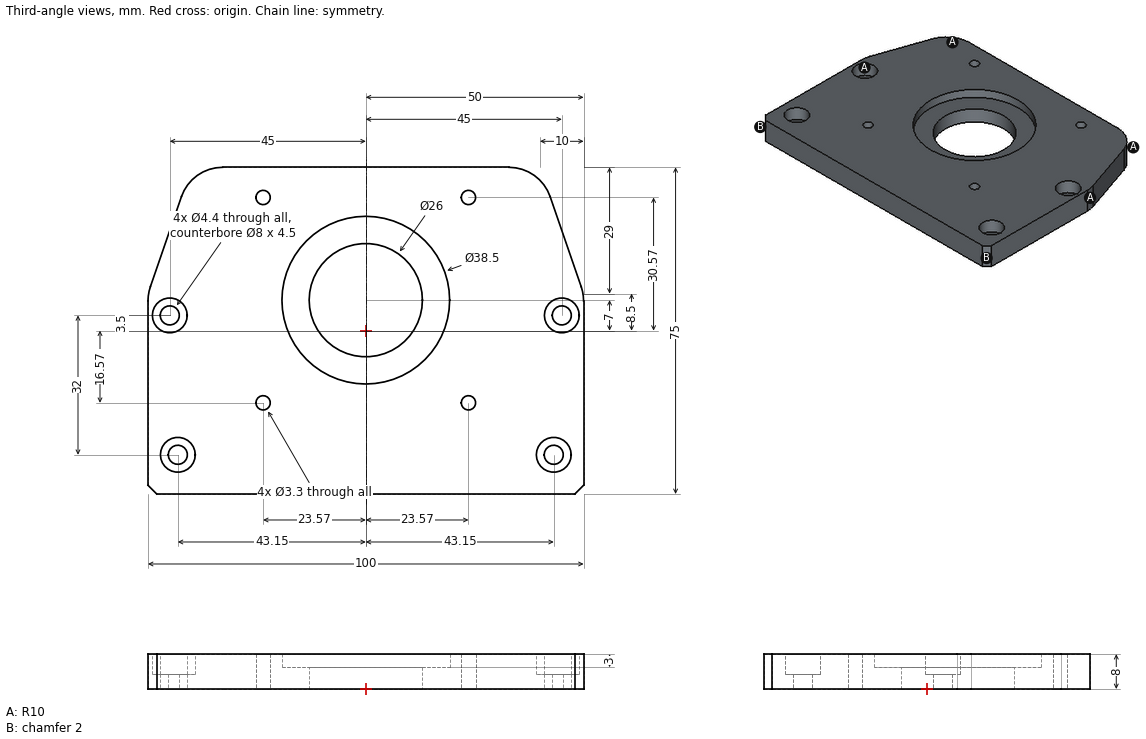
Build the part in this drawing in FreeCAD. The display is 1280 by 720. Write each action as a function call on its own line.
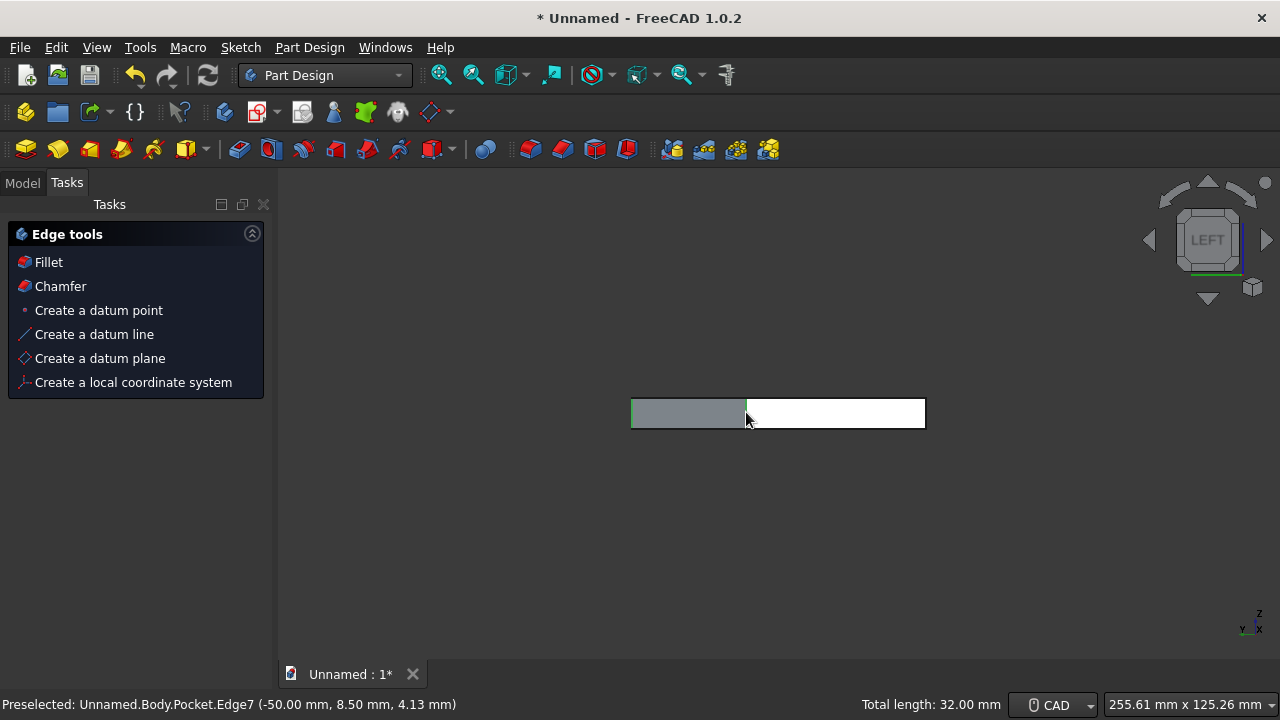
click(532, 150)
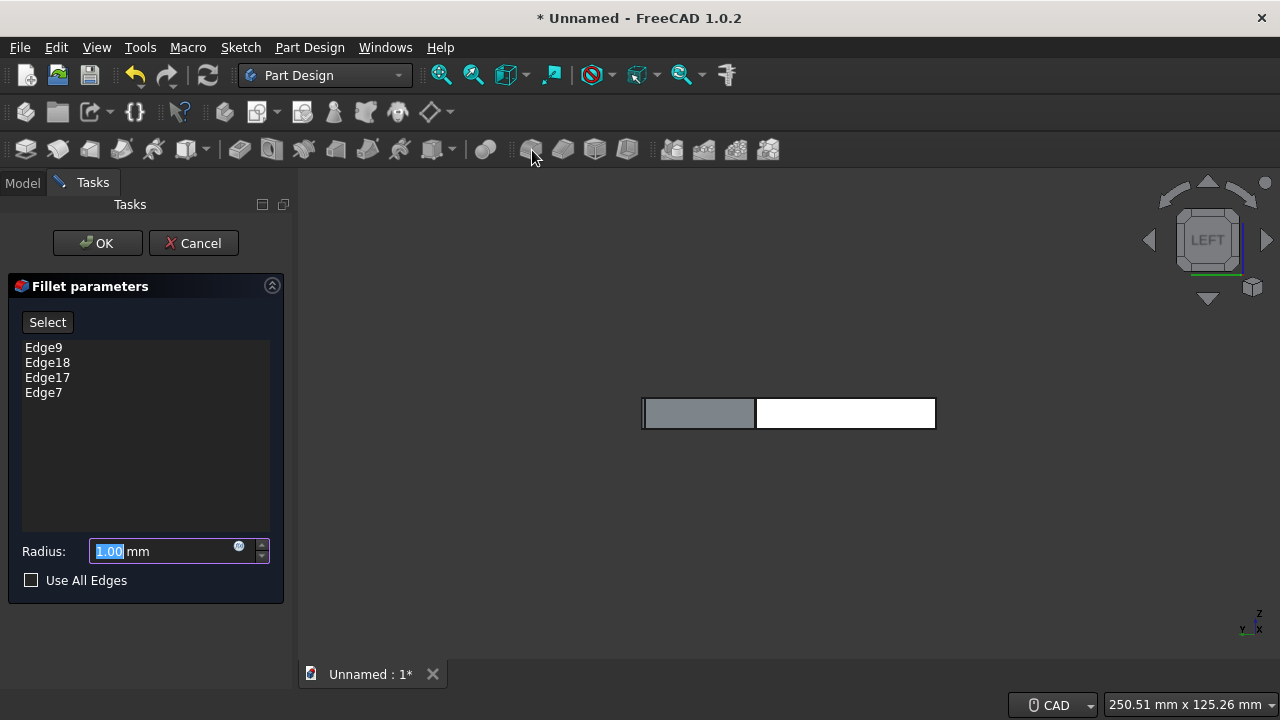
text(10)
key(Tab)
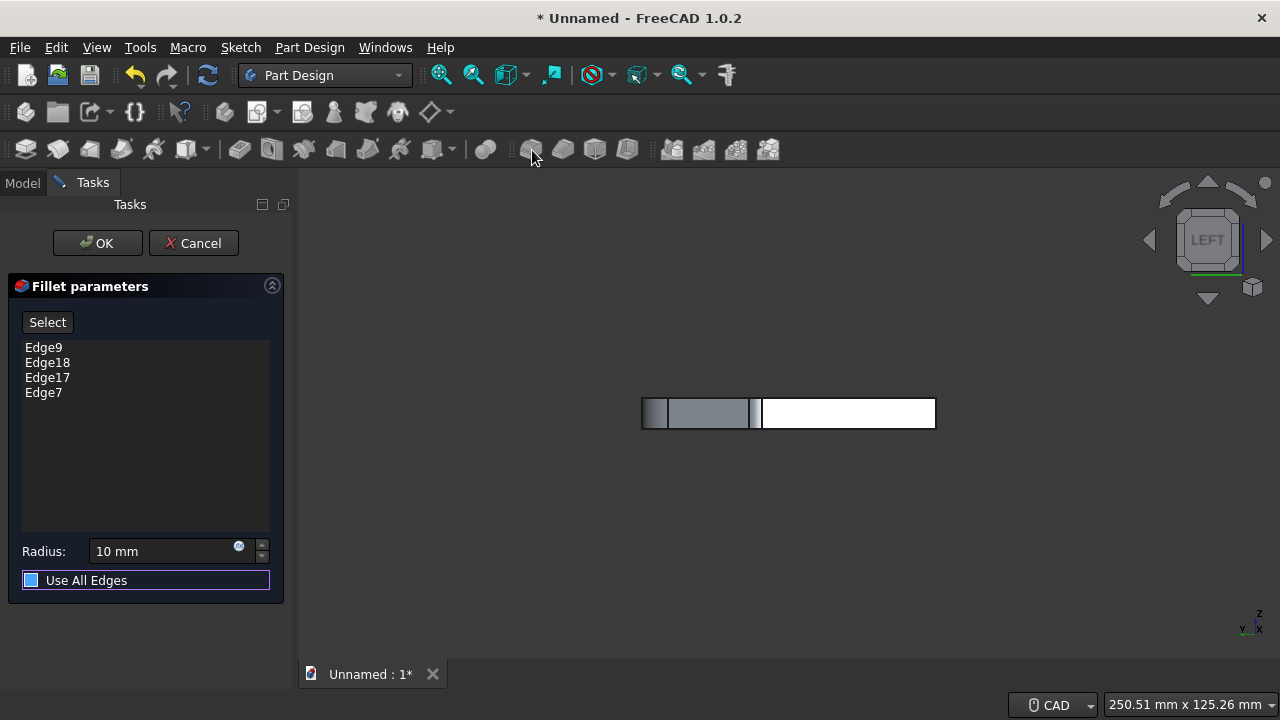
click(98, 243)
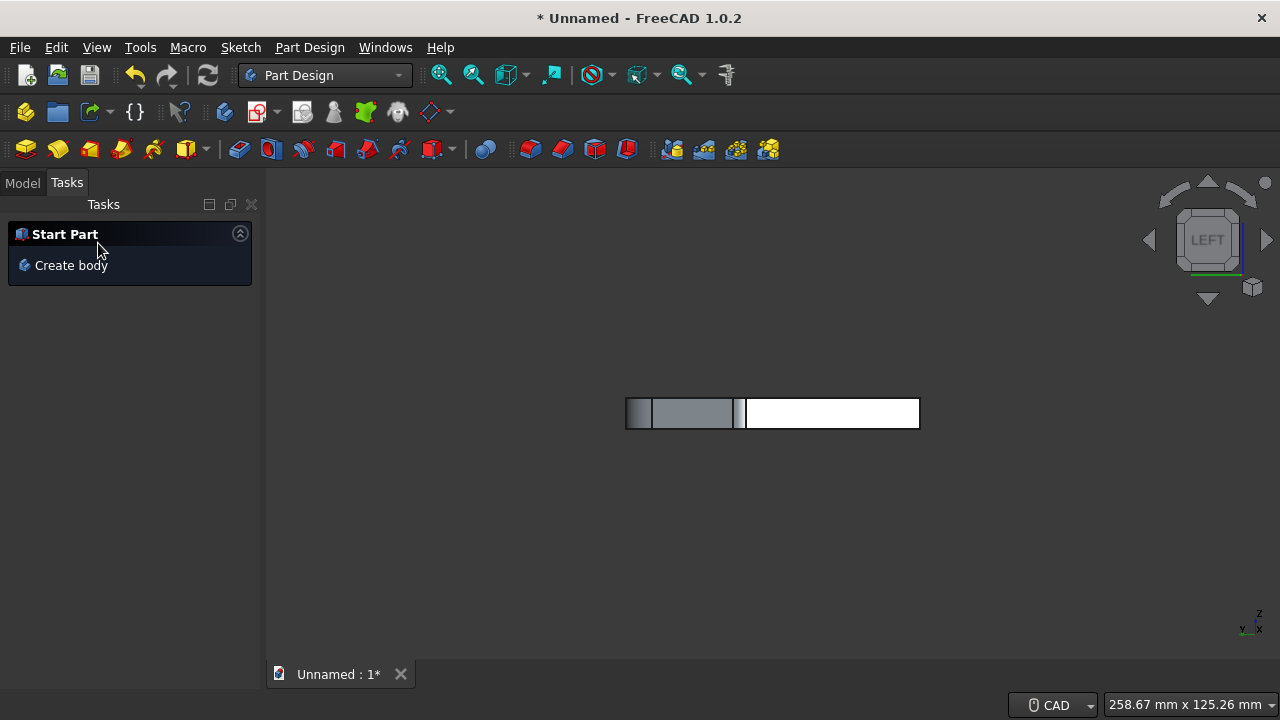
click(442, 76)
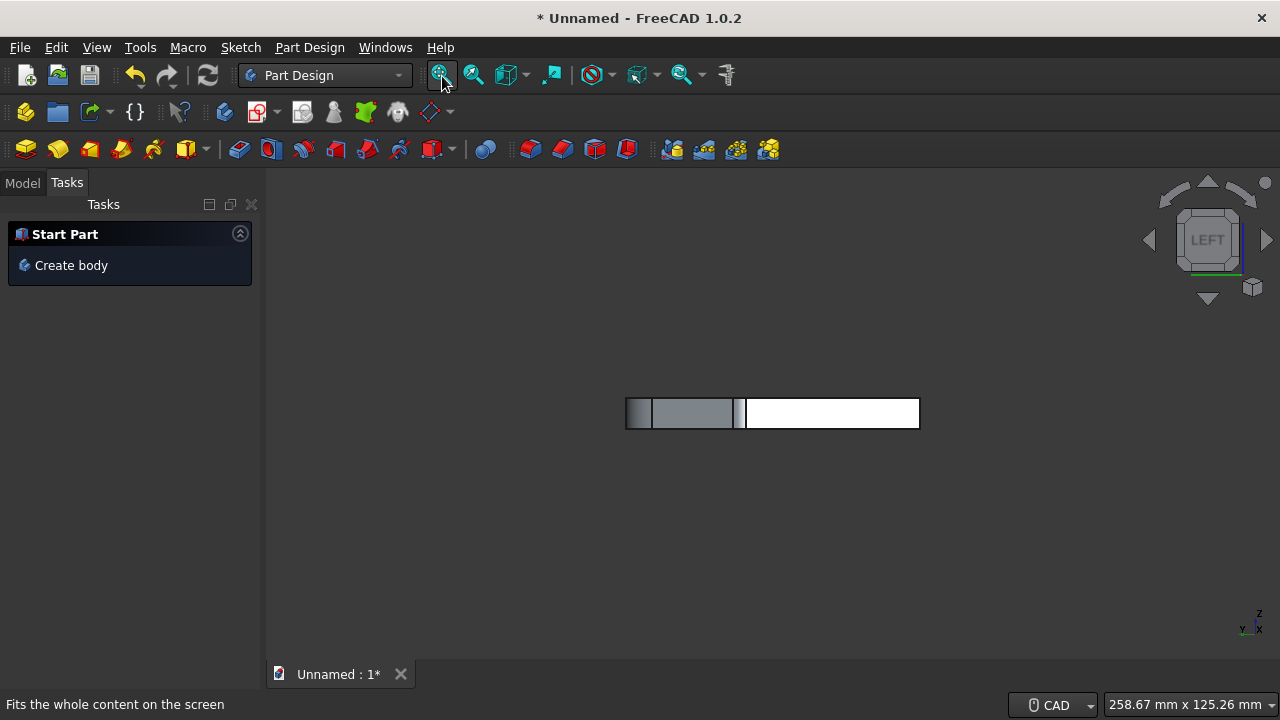
click(920, 412)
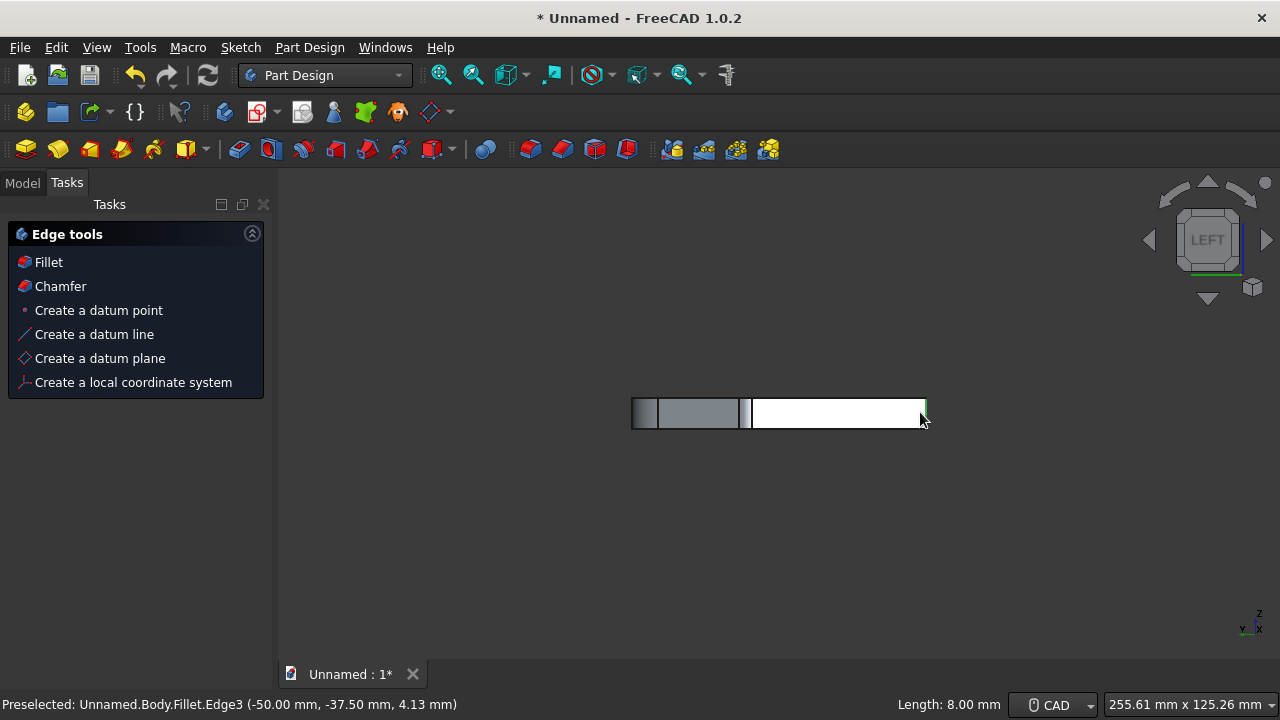
key(0)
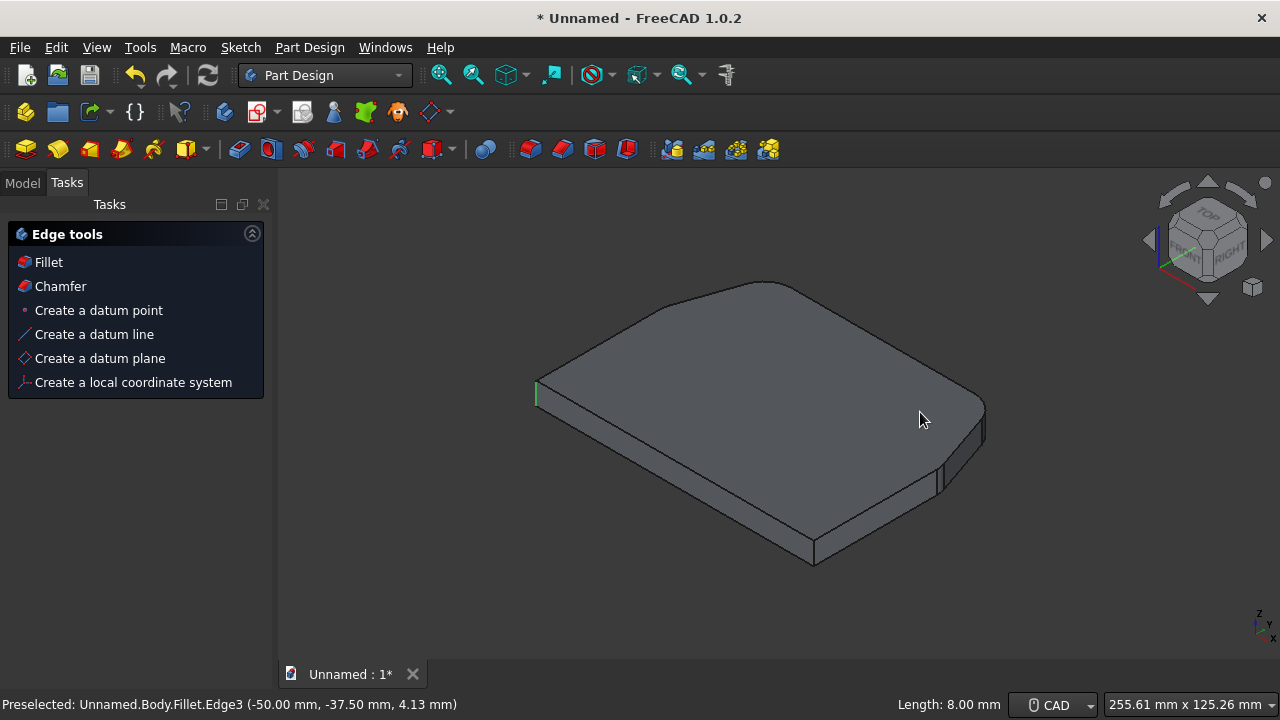
click(814, 553, ctrl)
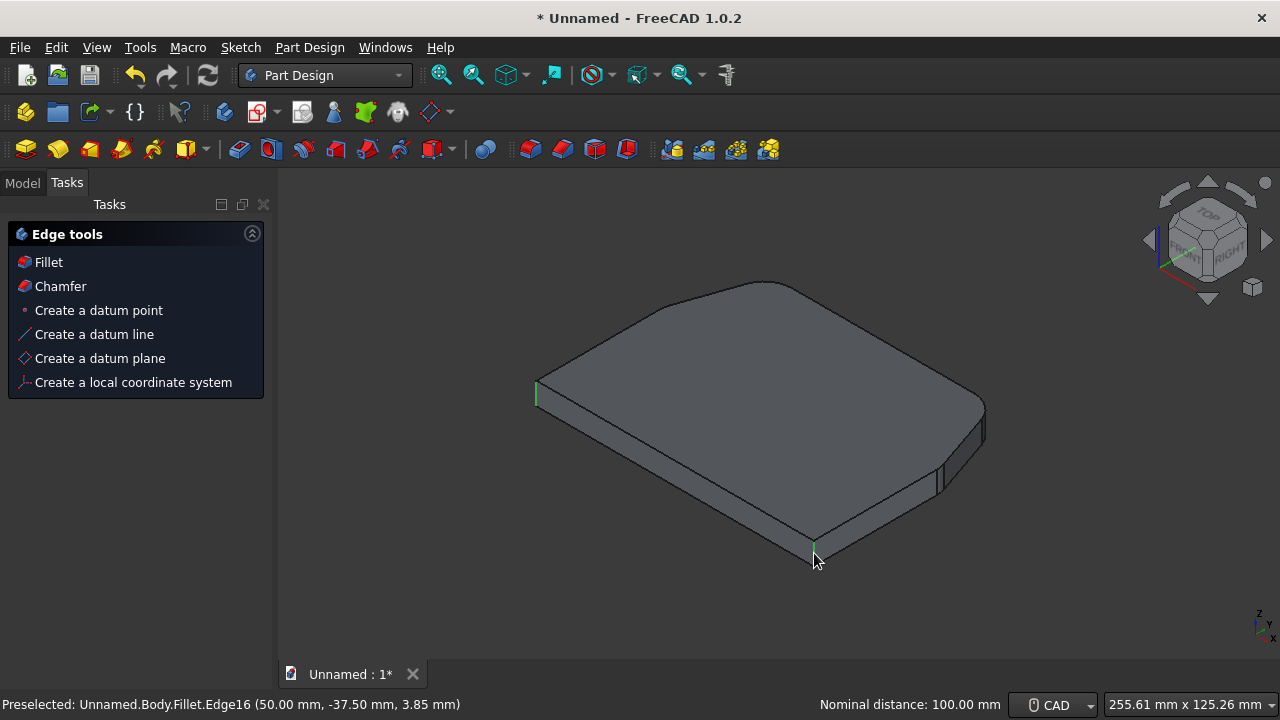
click(564, 150)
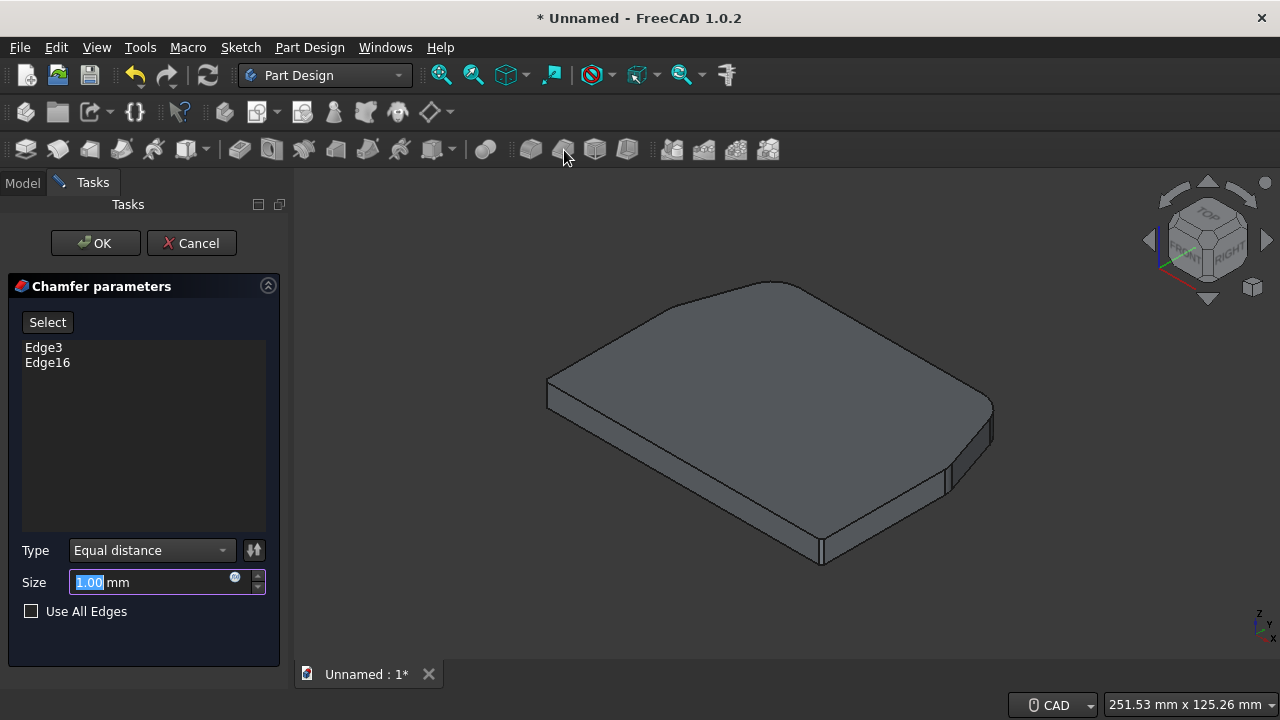
text(2)
key(Tab)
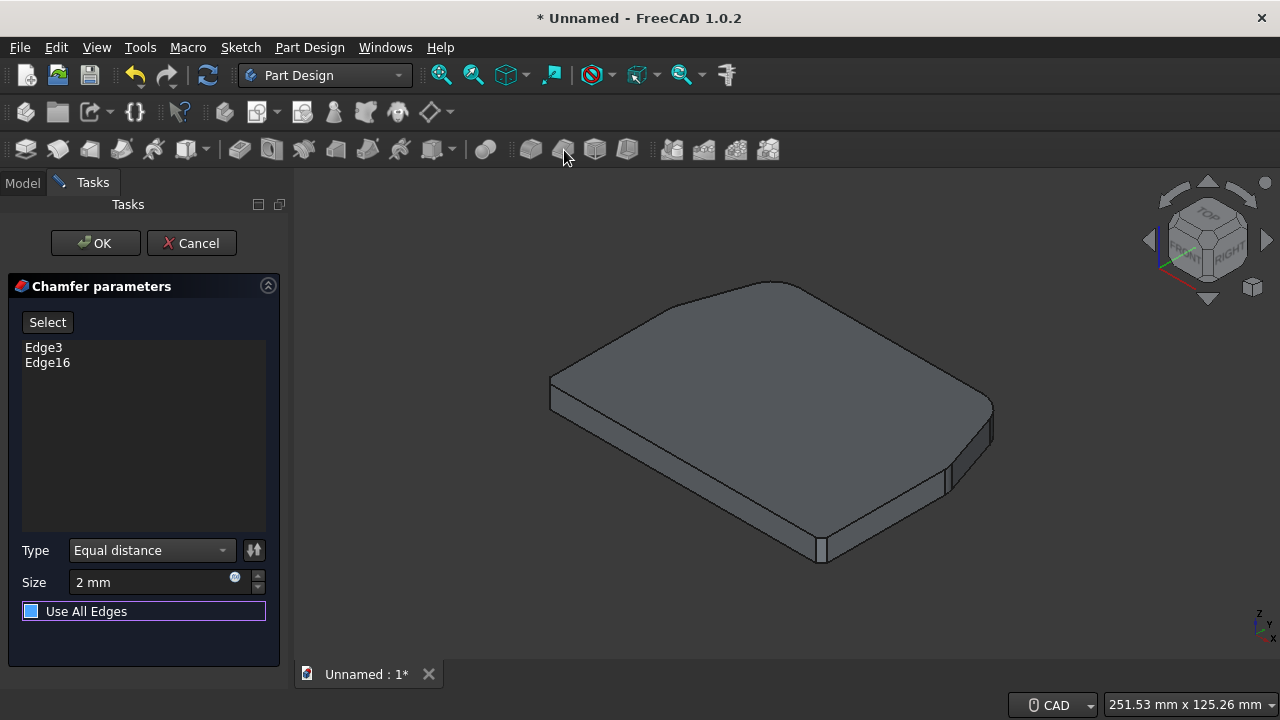
click(96, 243)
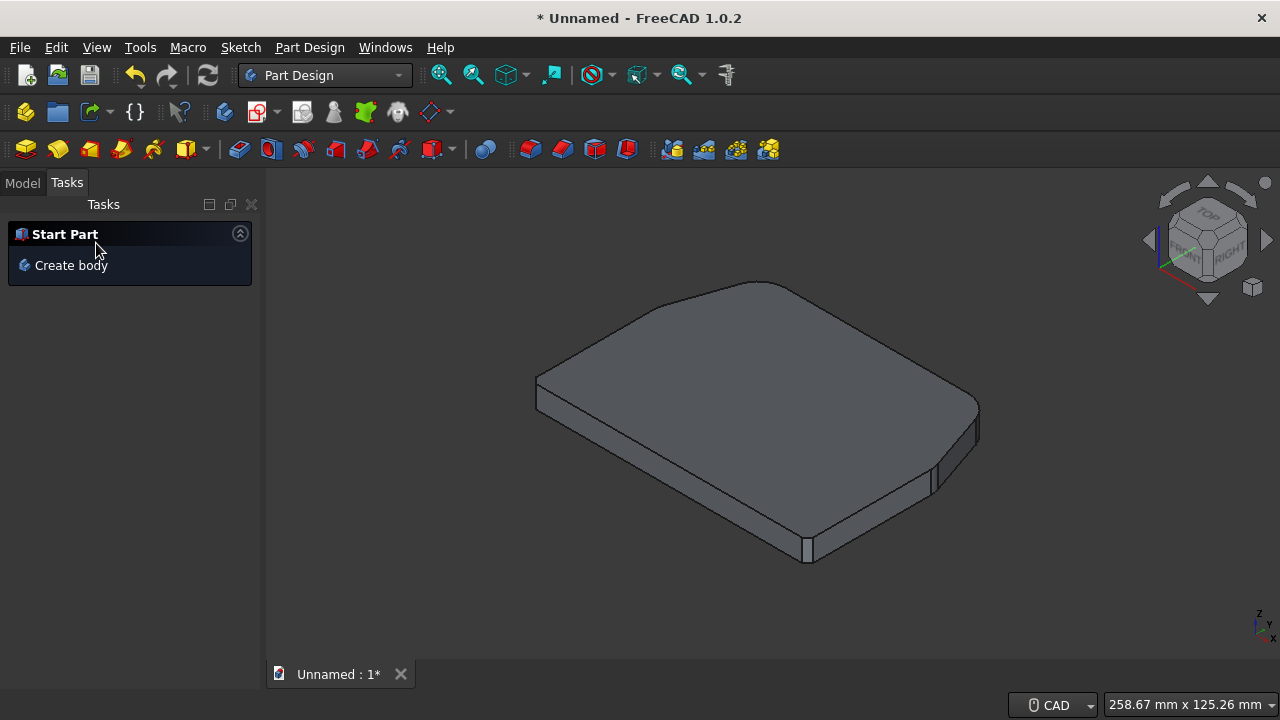
click(773, 400)